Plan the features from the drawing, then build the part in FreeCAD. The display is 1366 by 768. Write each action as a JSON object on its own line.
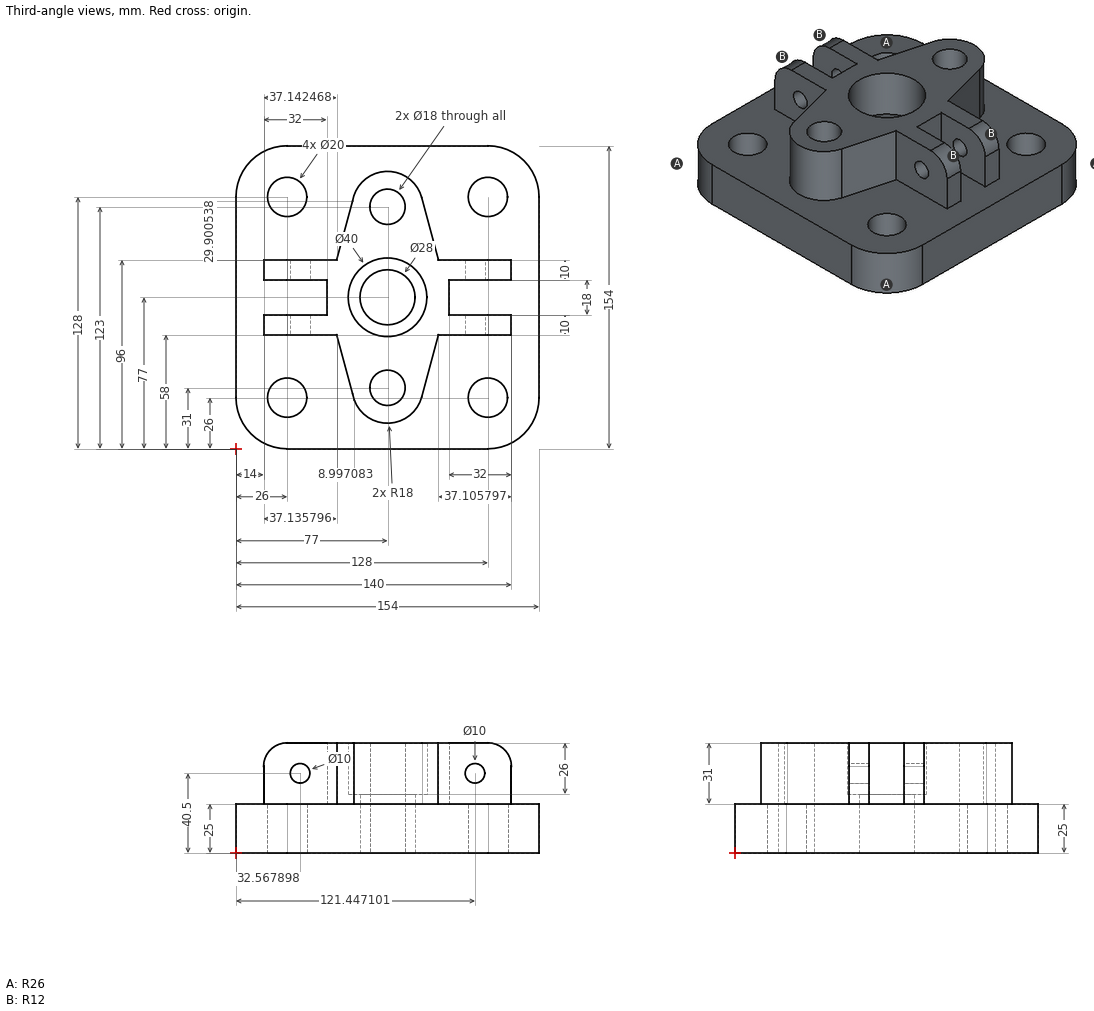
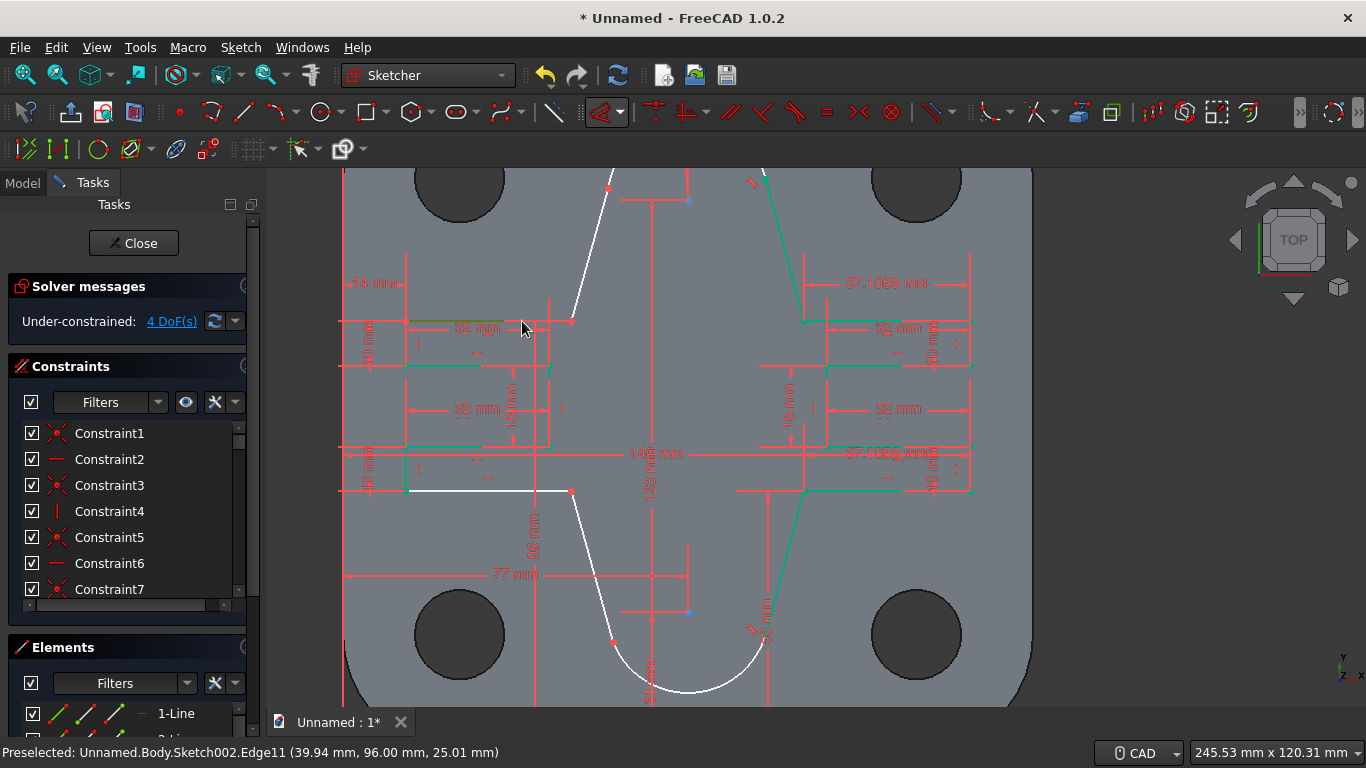
{"action": "key", "text": "l"}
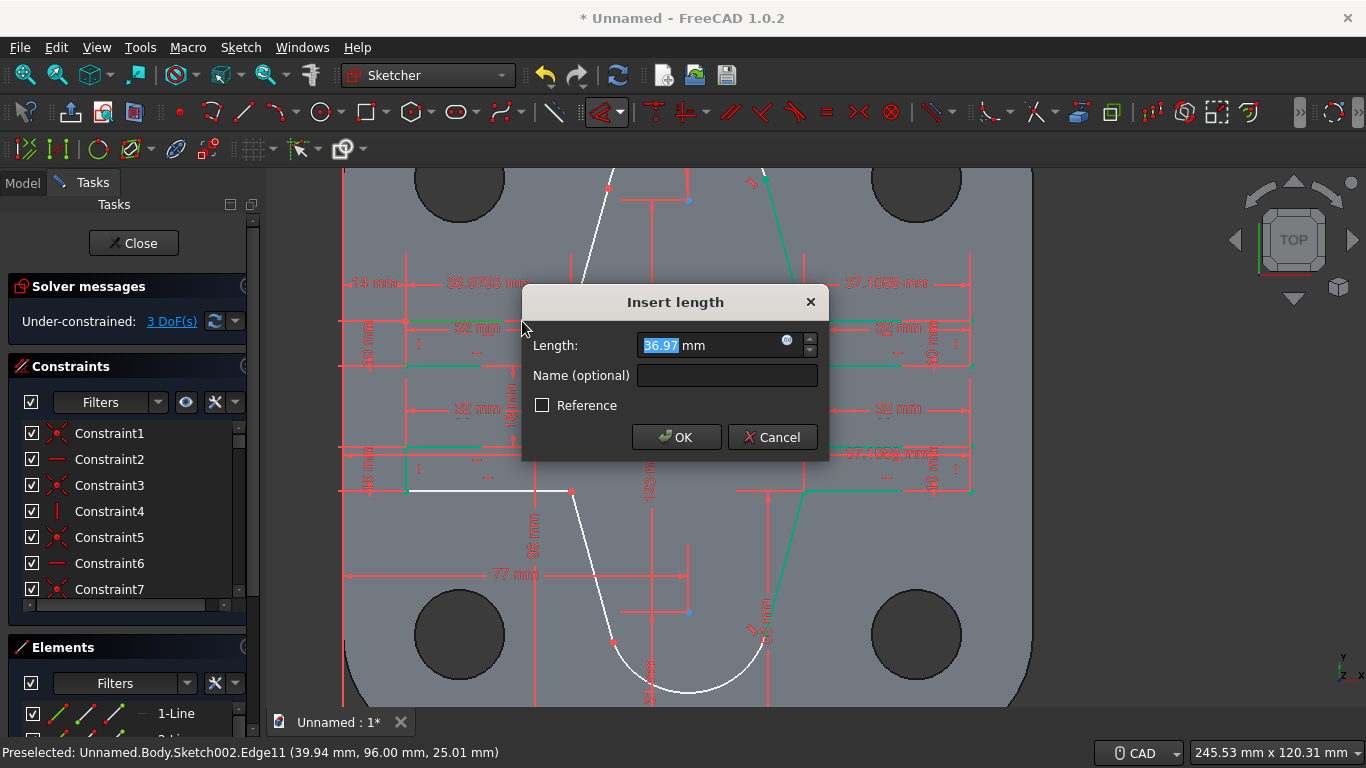
{"action": "type", "text": "37.142468"}
{"action": "key", "text": "Return"}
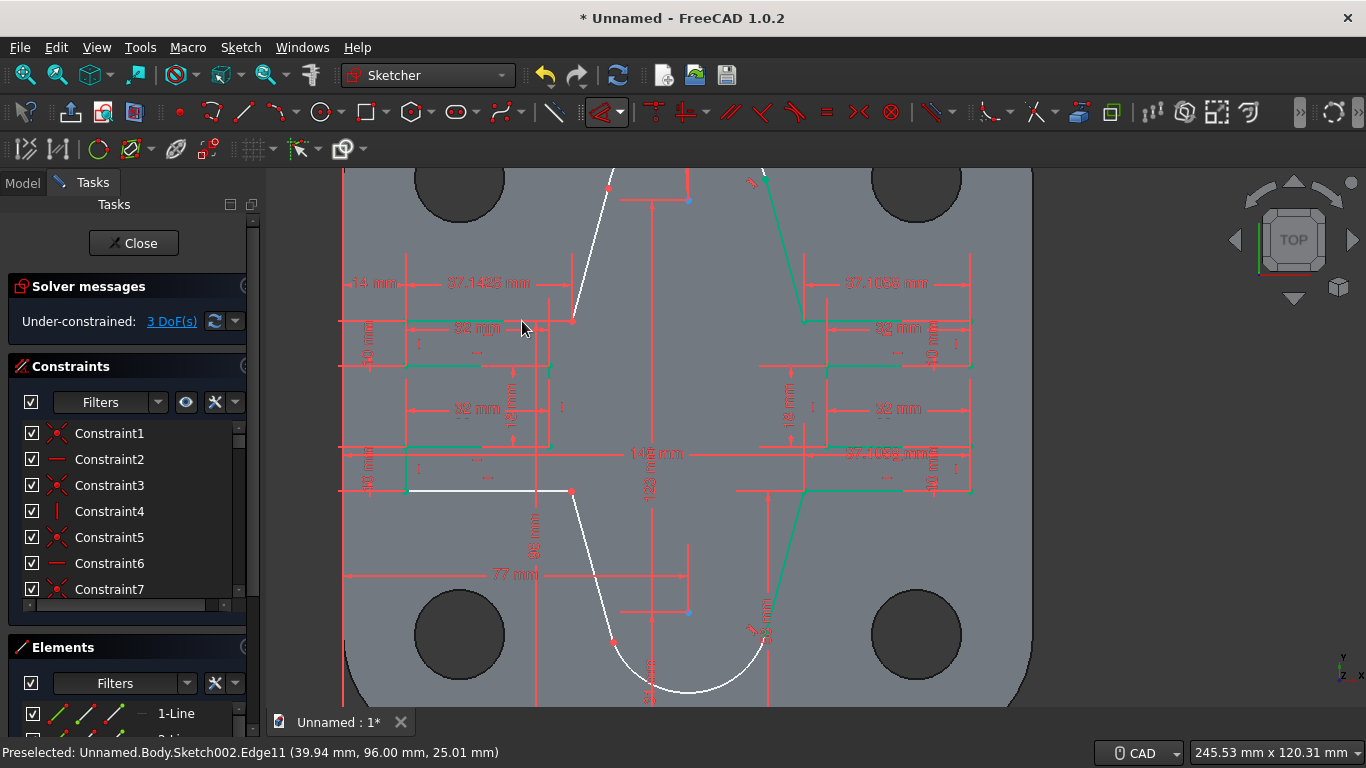
{"action": "left_click", "coordinate": [455, 491]}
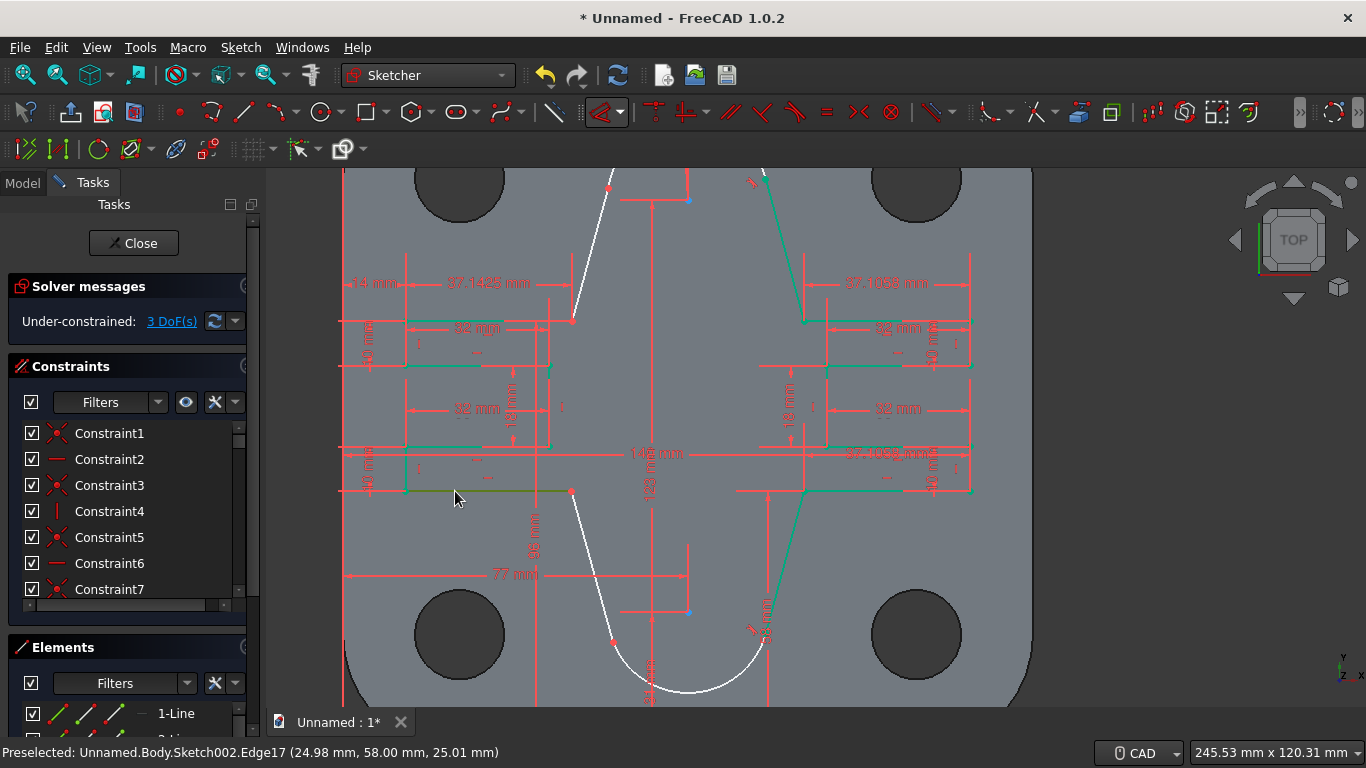
{"action": "left_click", "coordinate": [622, 112]}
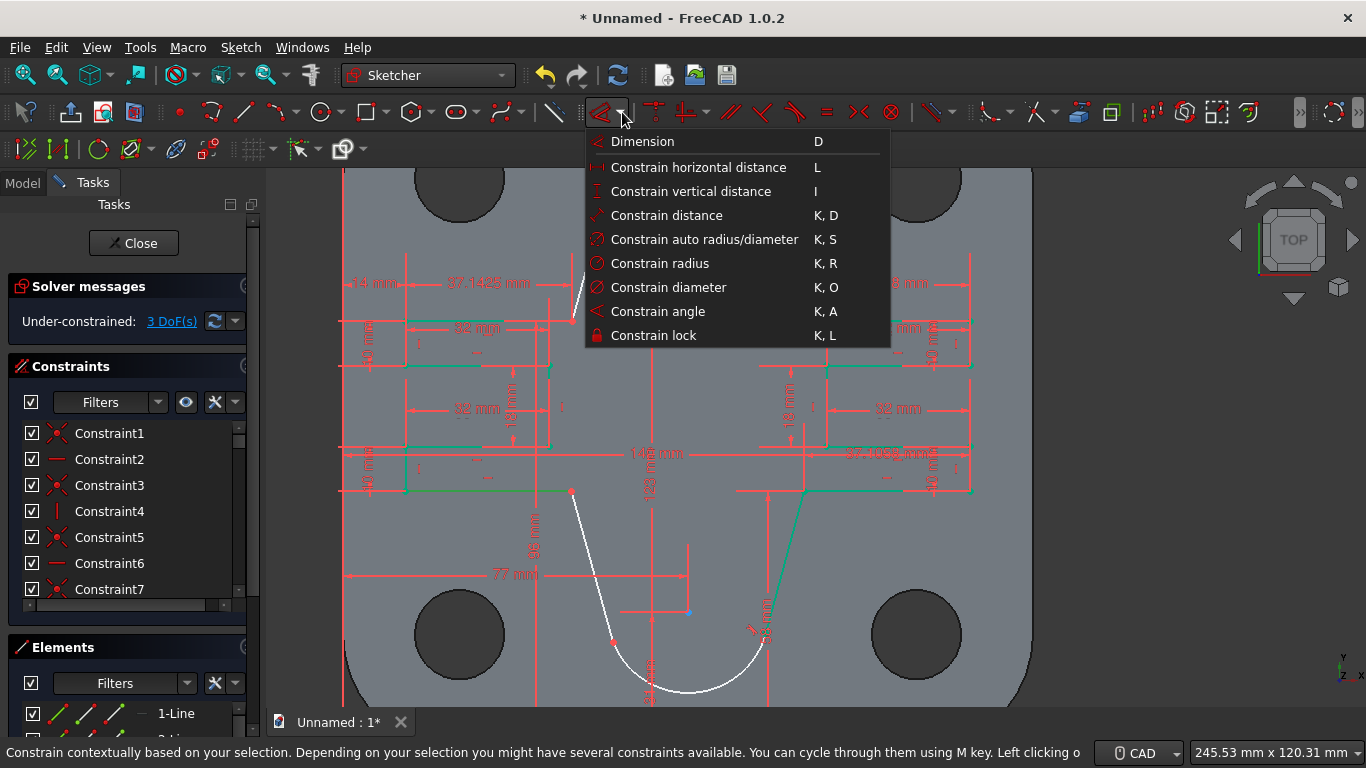
{"action": "left_click", "coordinate": [738, 167]}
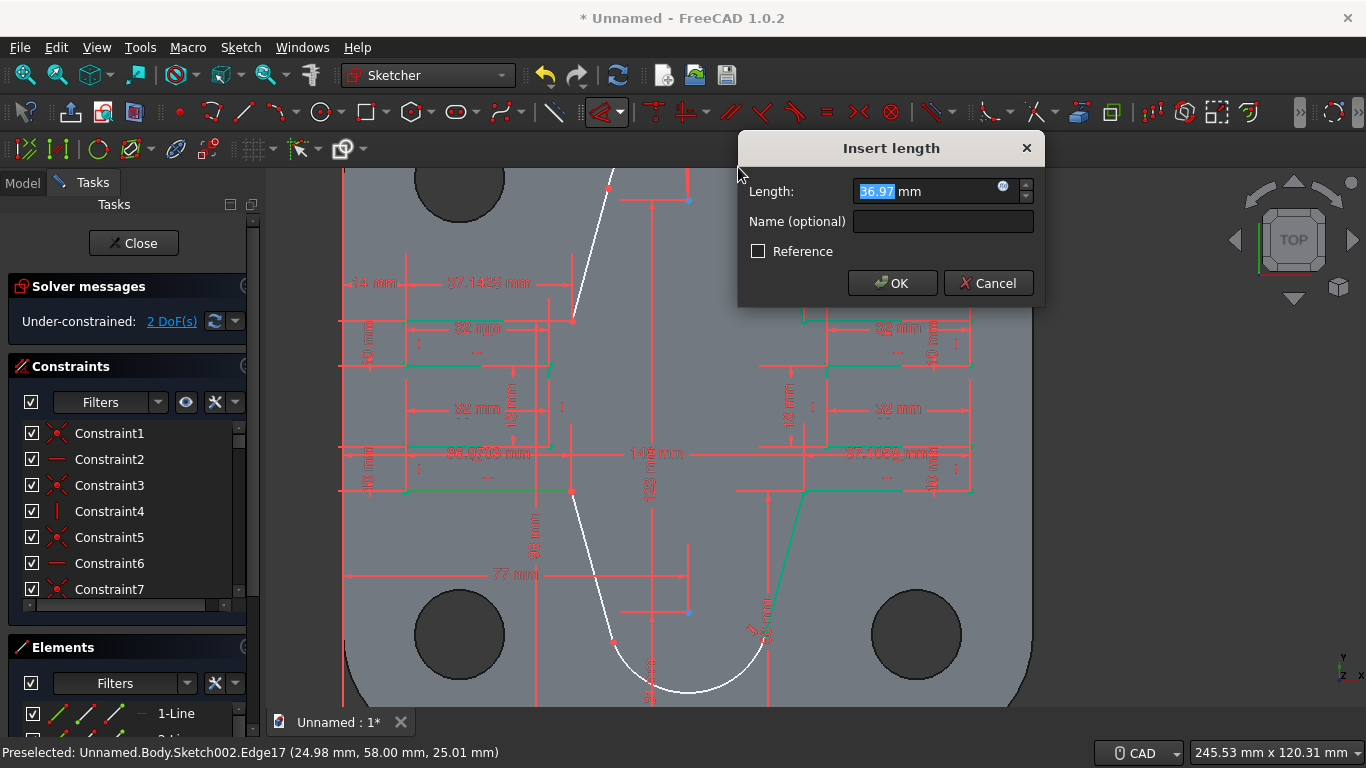
{"action": "type", "text": "37.135796"}
{"action": "key", "text": "Return"}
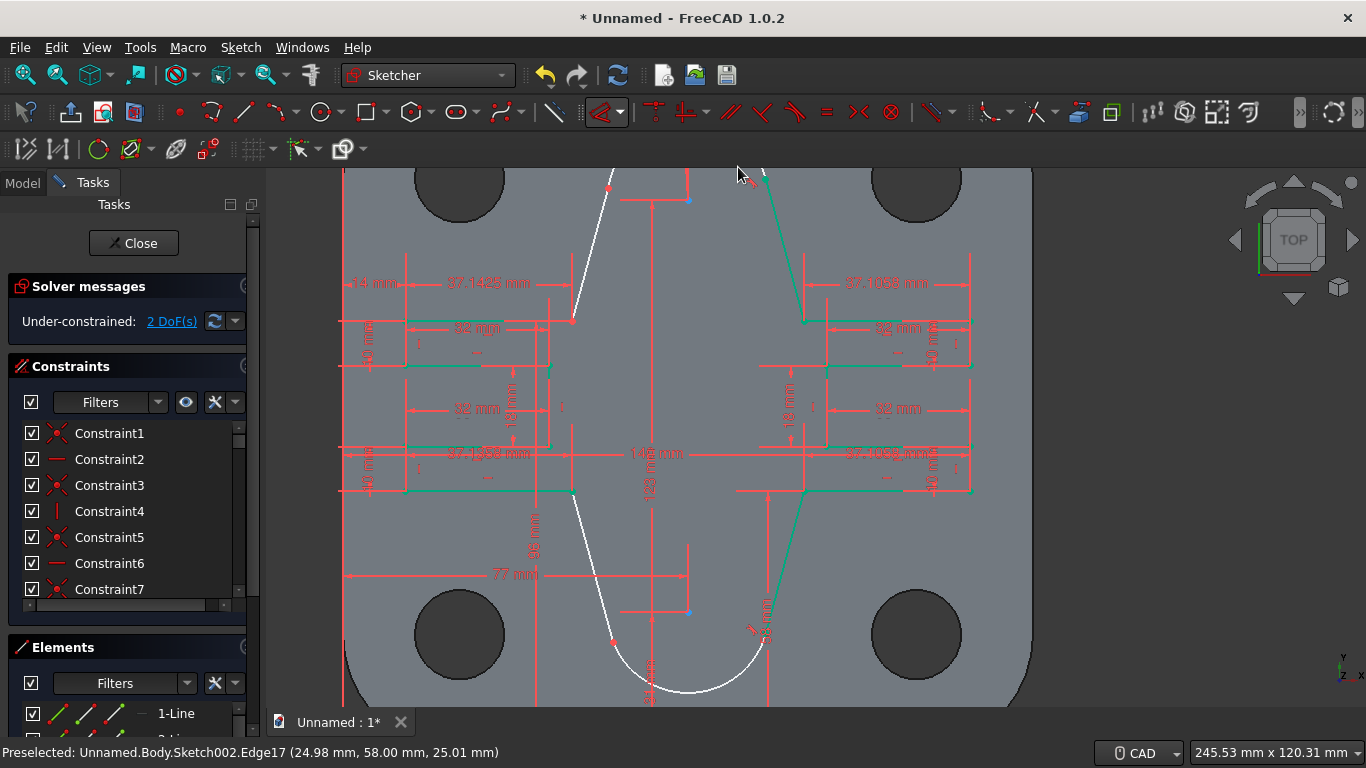
{"action": "left_click", "coordinate": [584, 537]}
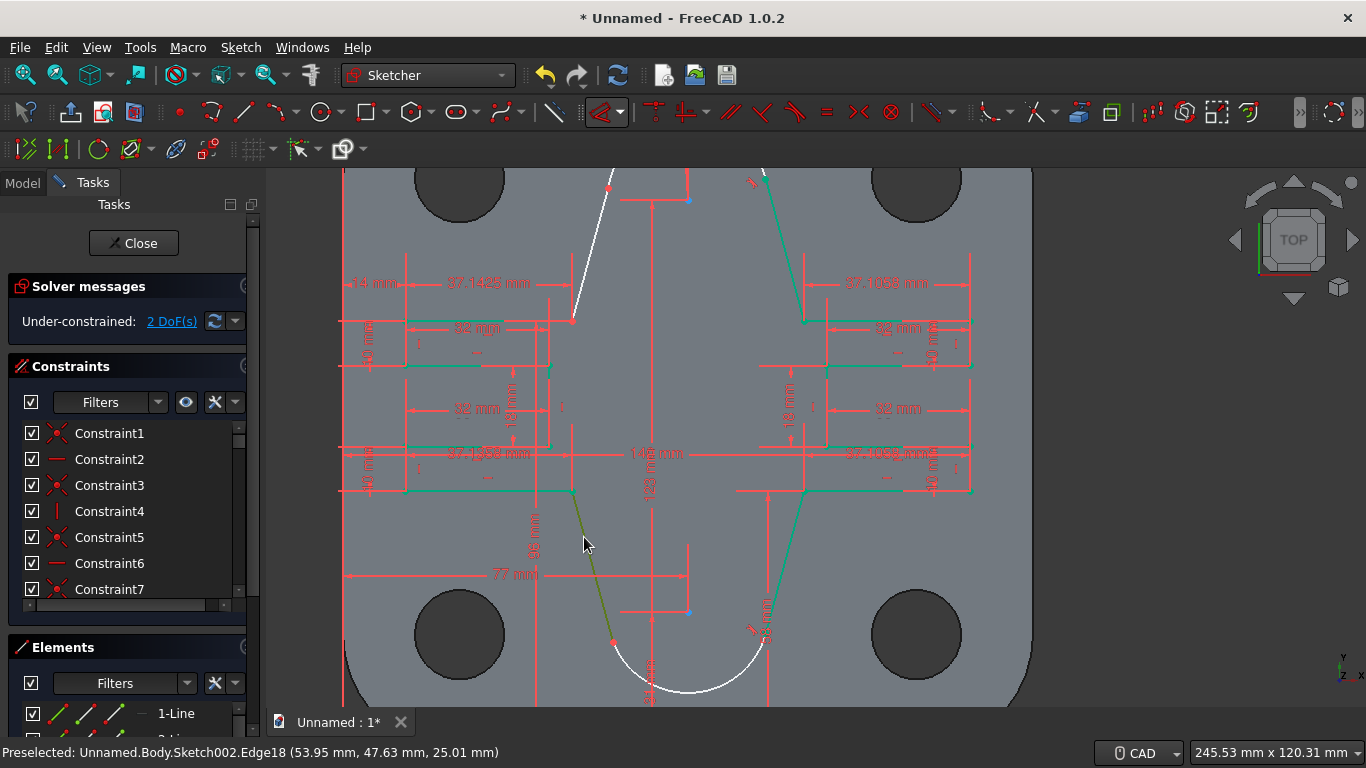
{"action": "key", "text": "l"}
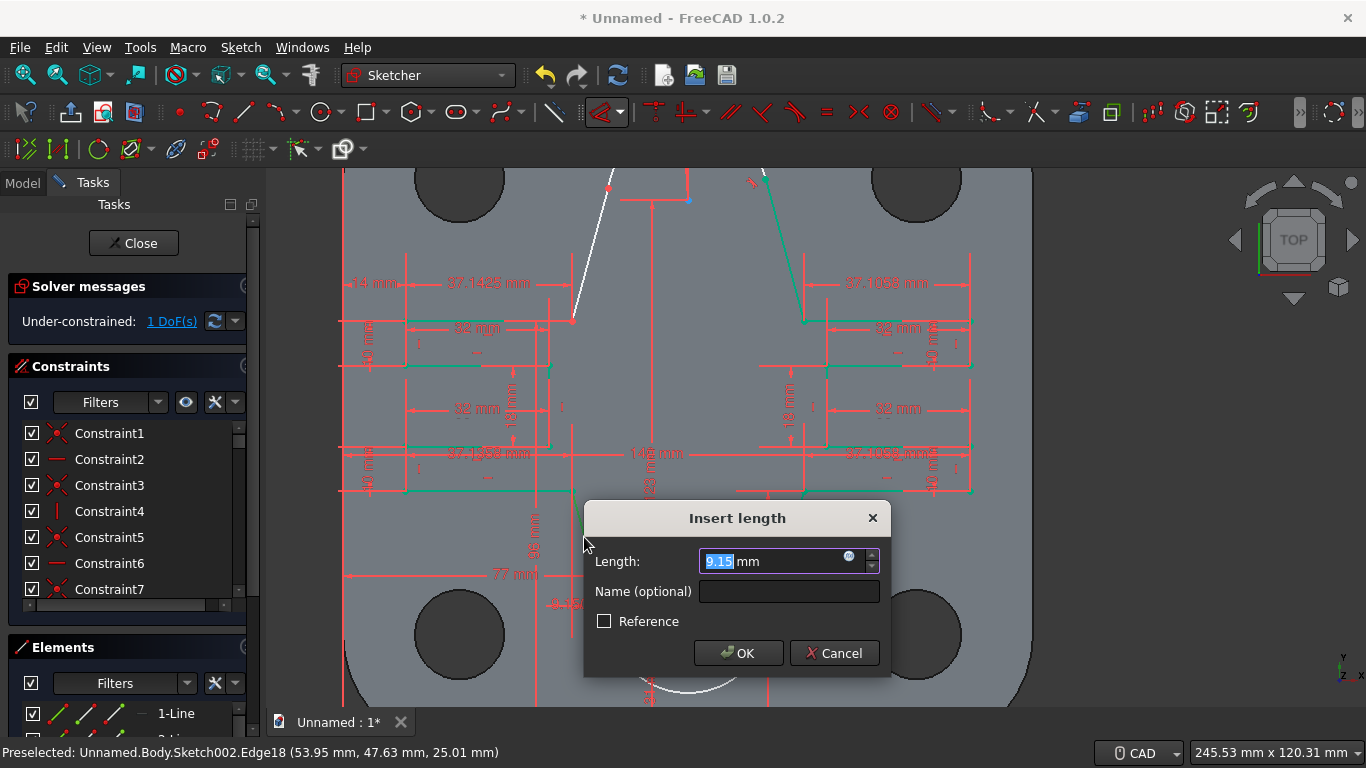
{"action": "type", "text": "8.997083"}
{"action": "key", "text": "Return"}